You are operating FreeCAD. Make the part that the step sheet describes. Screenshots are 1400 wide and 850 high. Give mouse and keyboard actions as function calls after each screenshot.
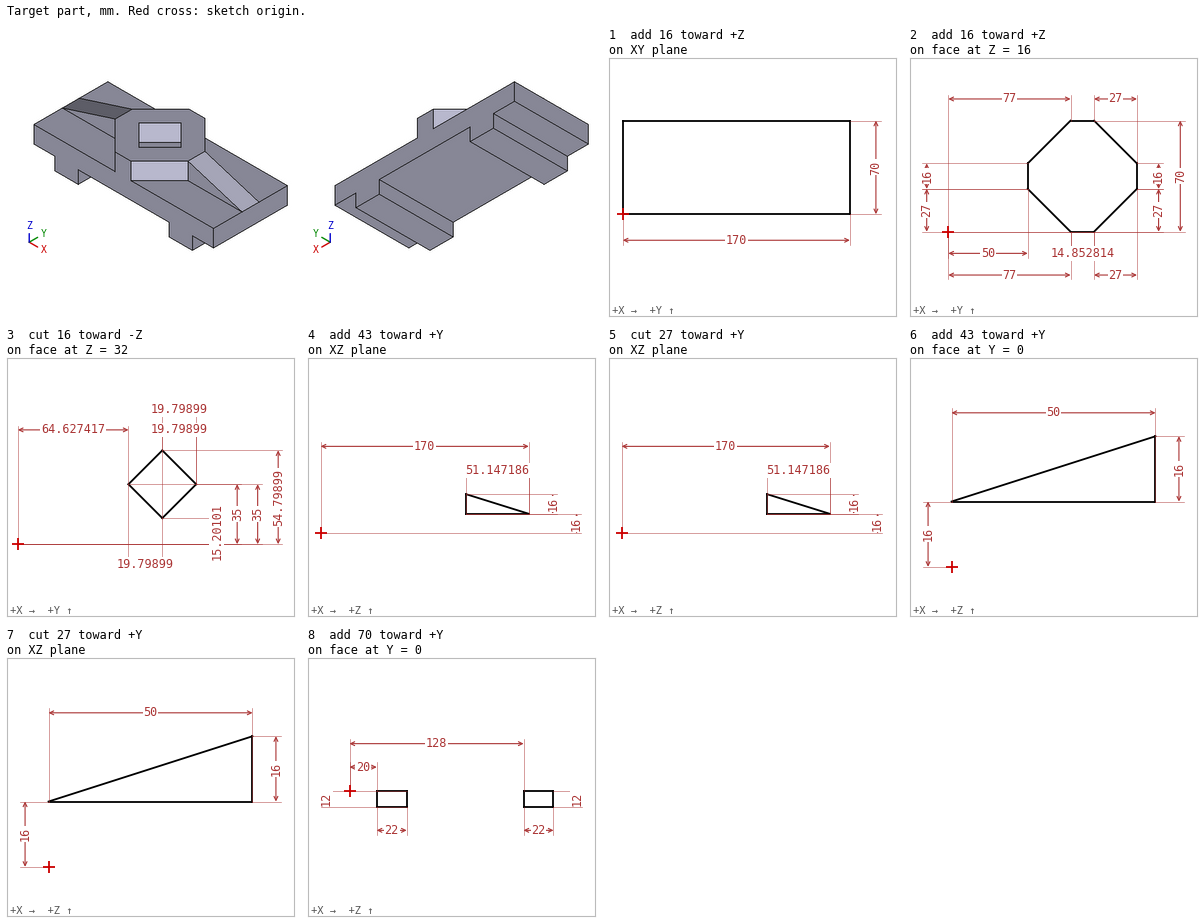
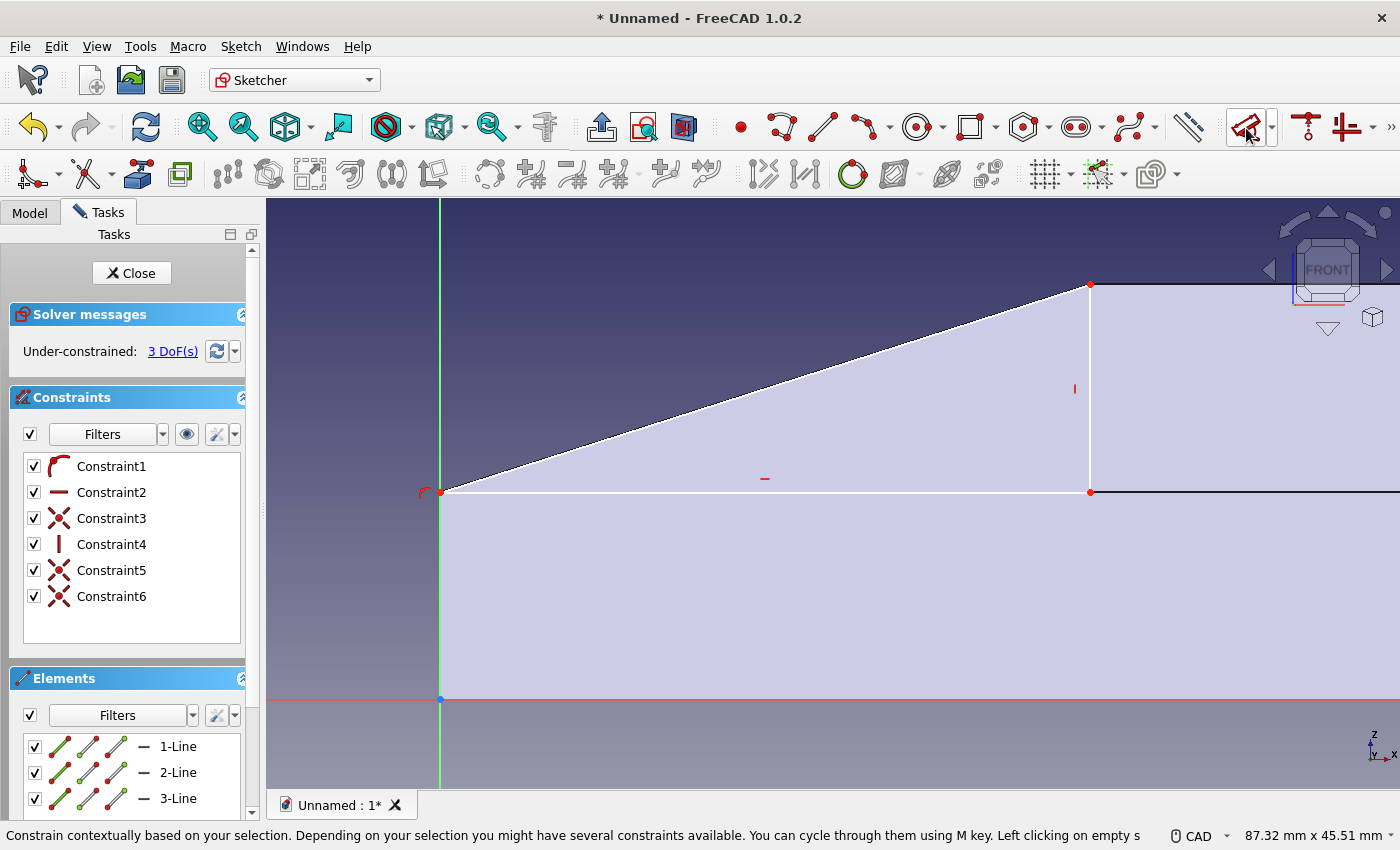
click(635, 493)
click(765, 527)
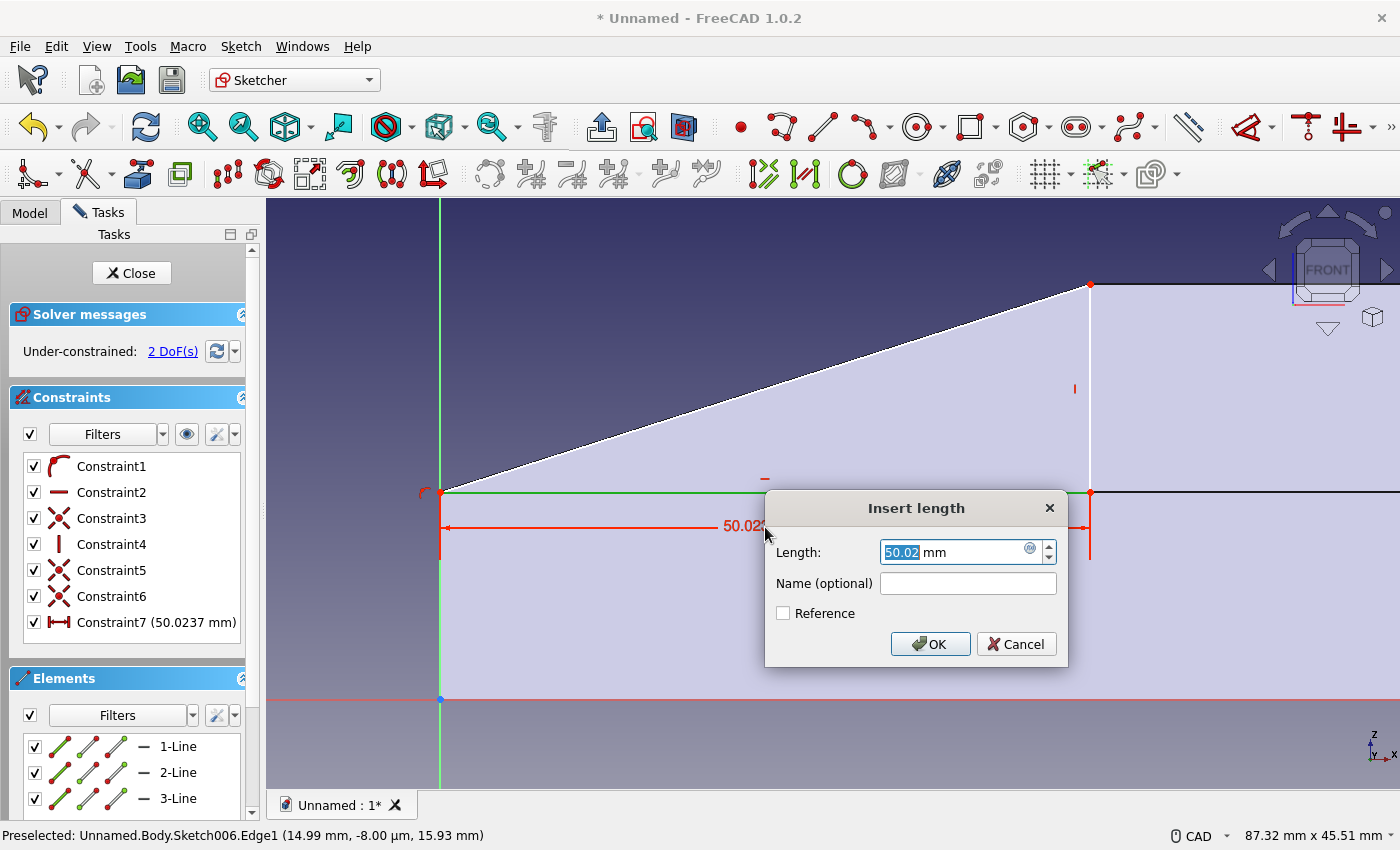
text(50)
key(Return)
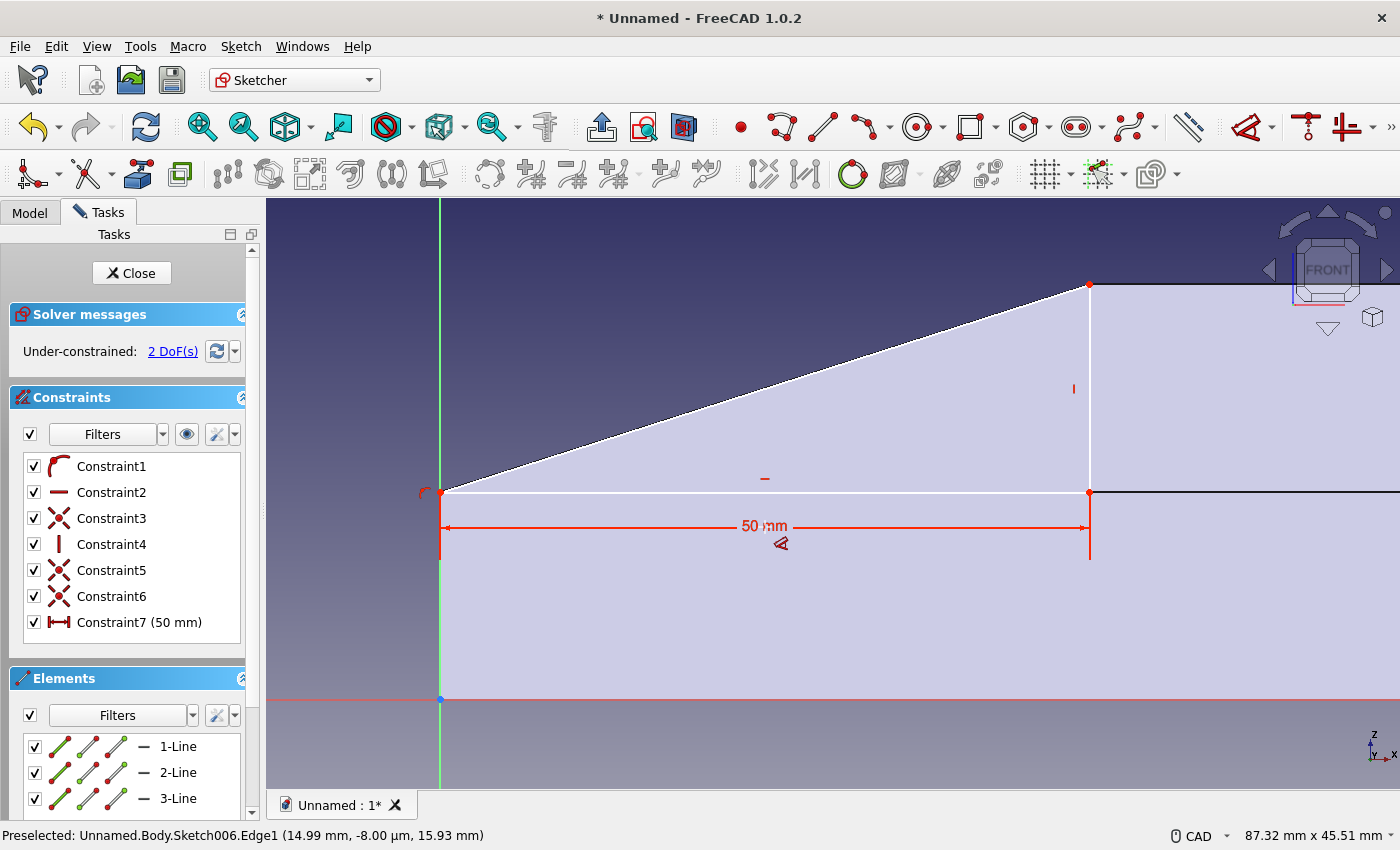
click(1090, 431)
click(1124, 389)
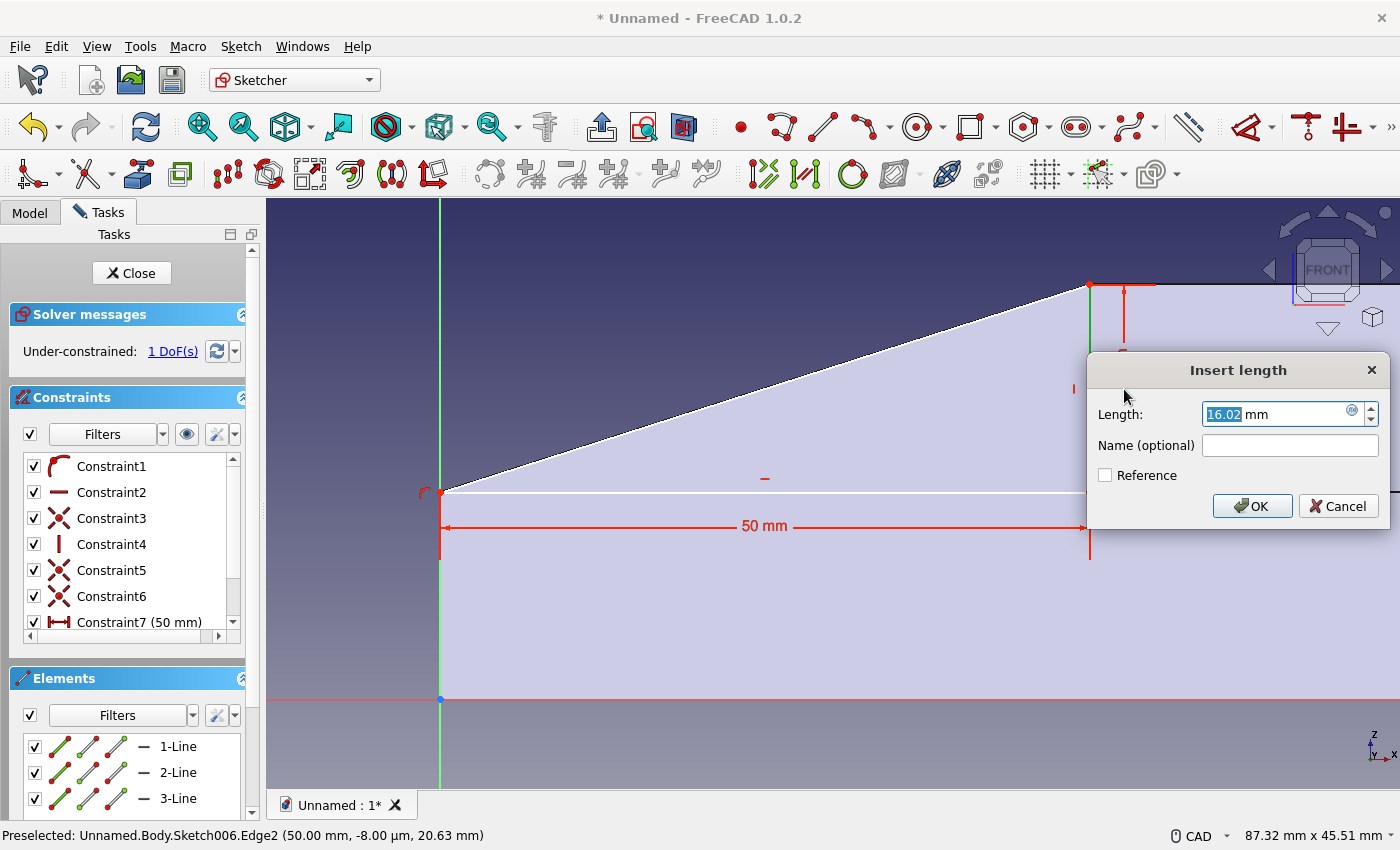
text(16)
key(Return)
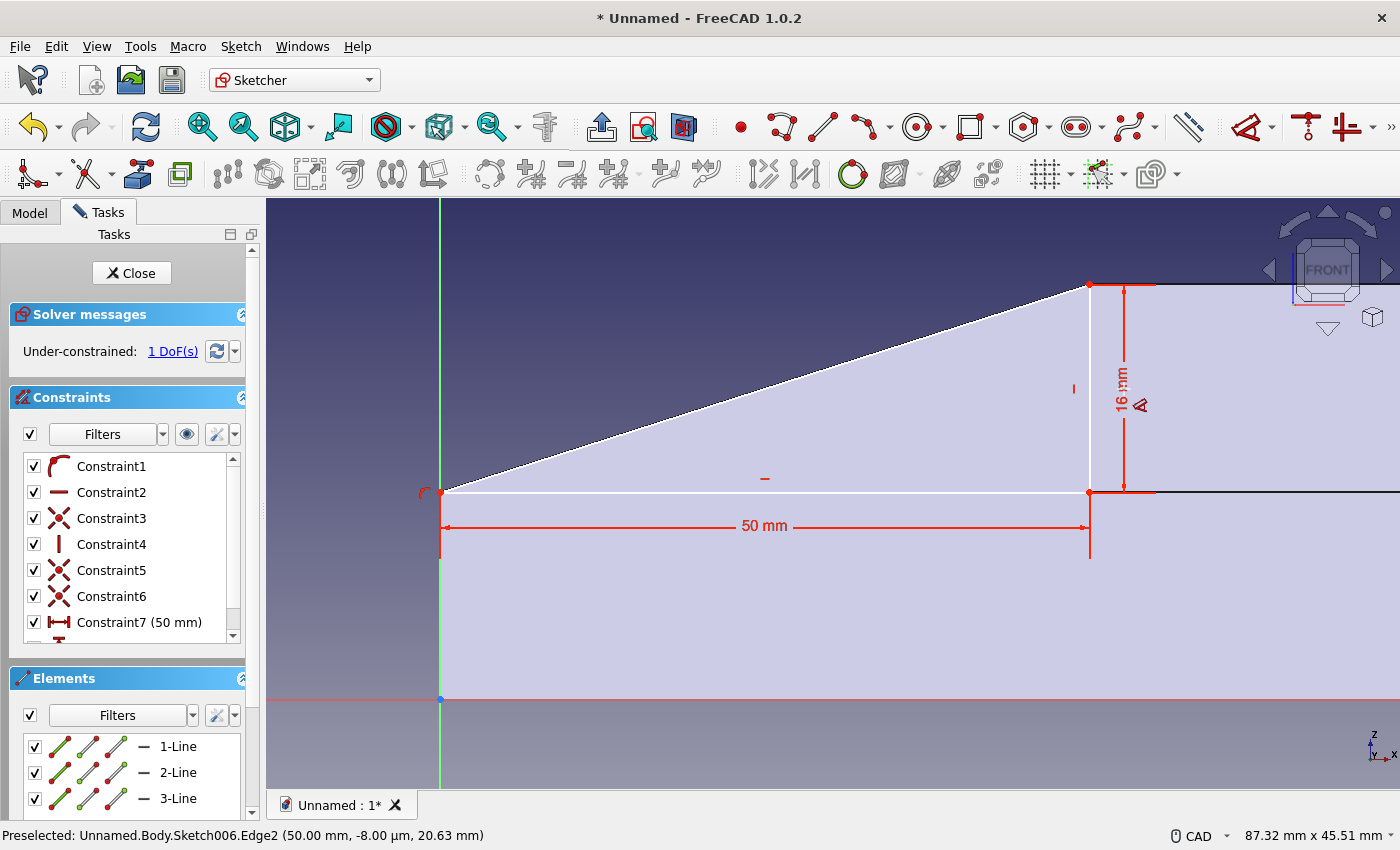
click(440, 493)
click(406, 596)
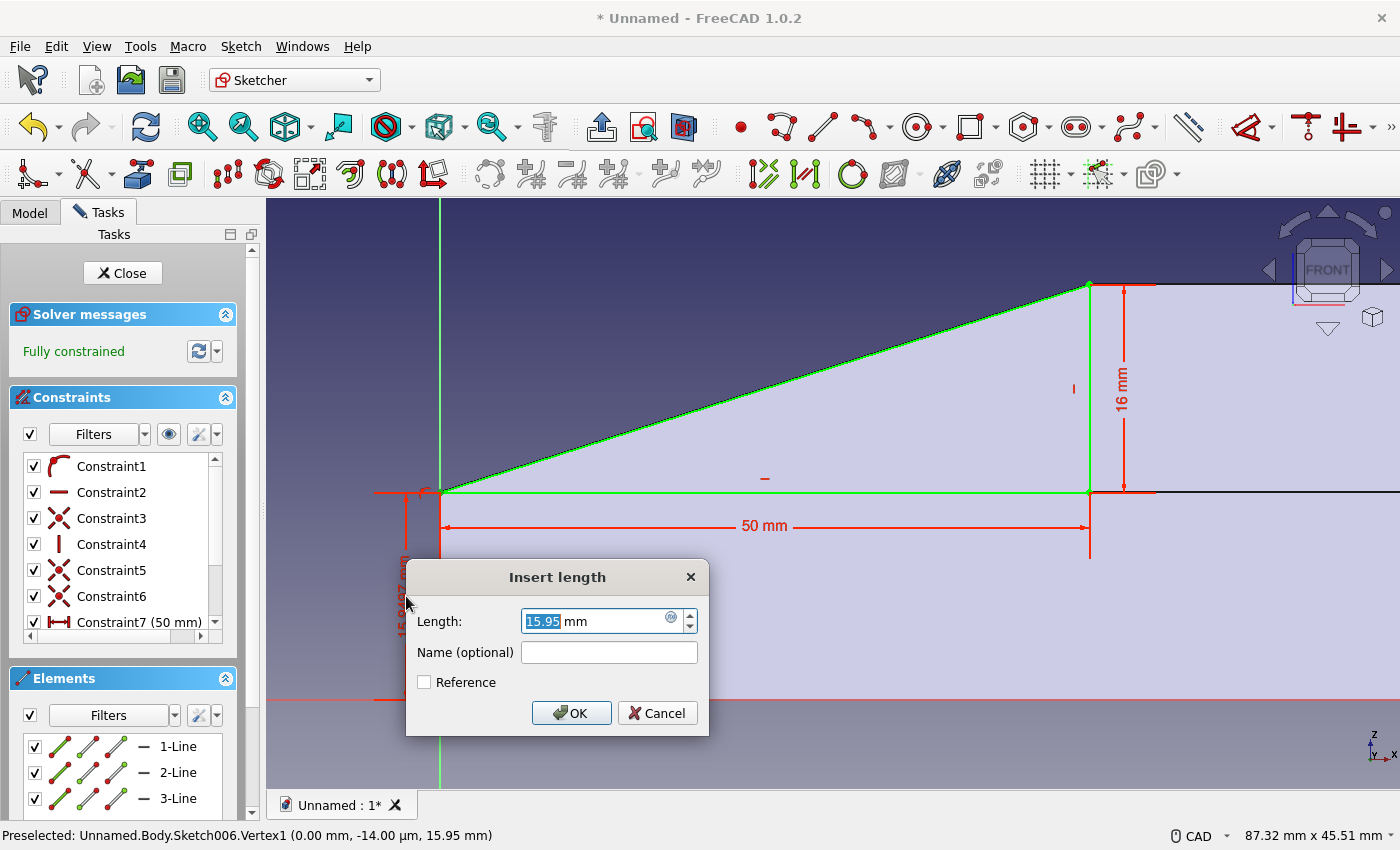
text(16)
key(Return)
key(Escape)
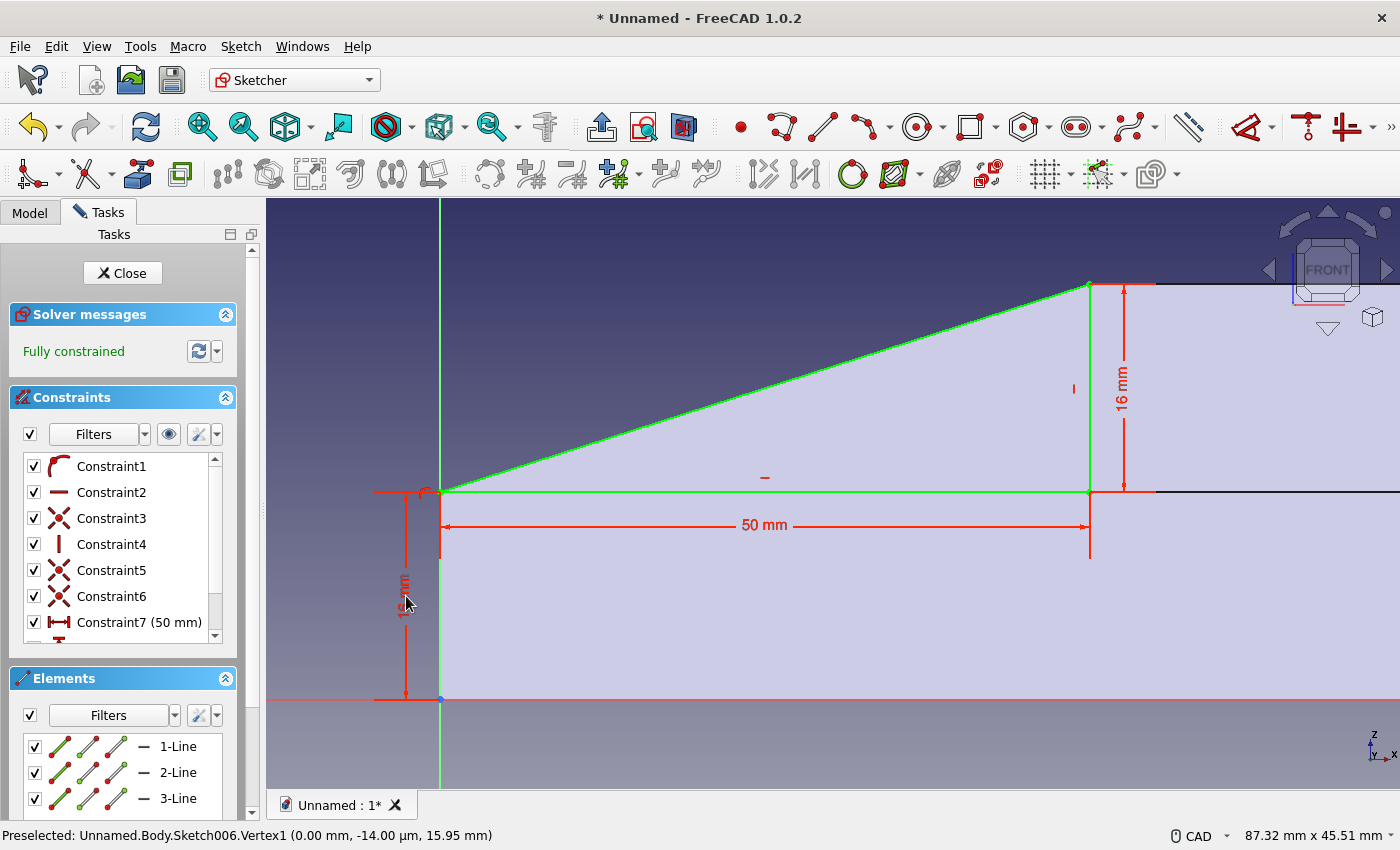
click(123, 273)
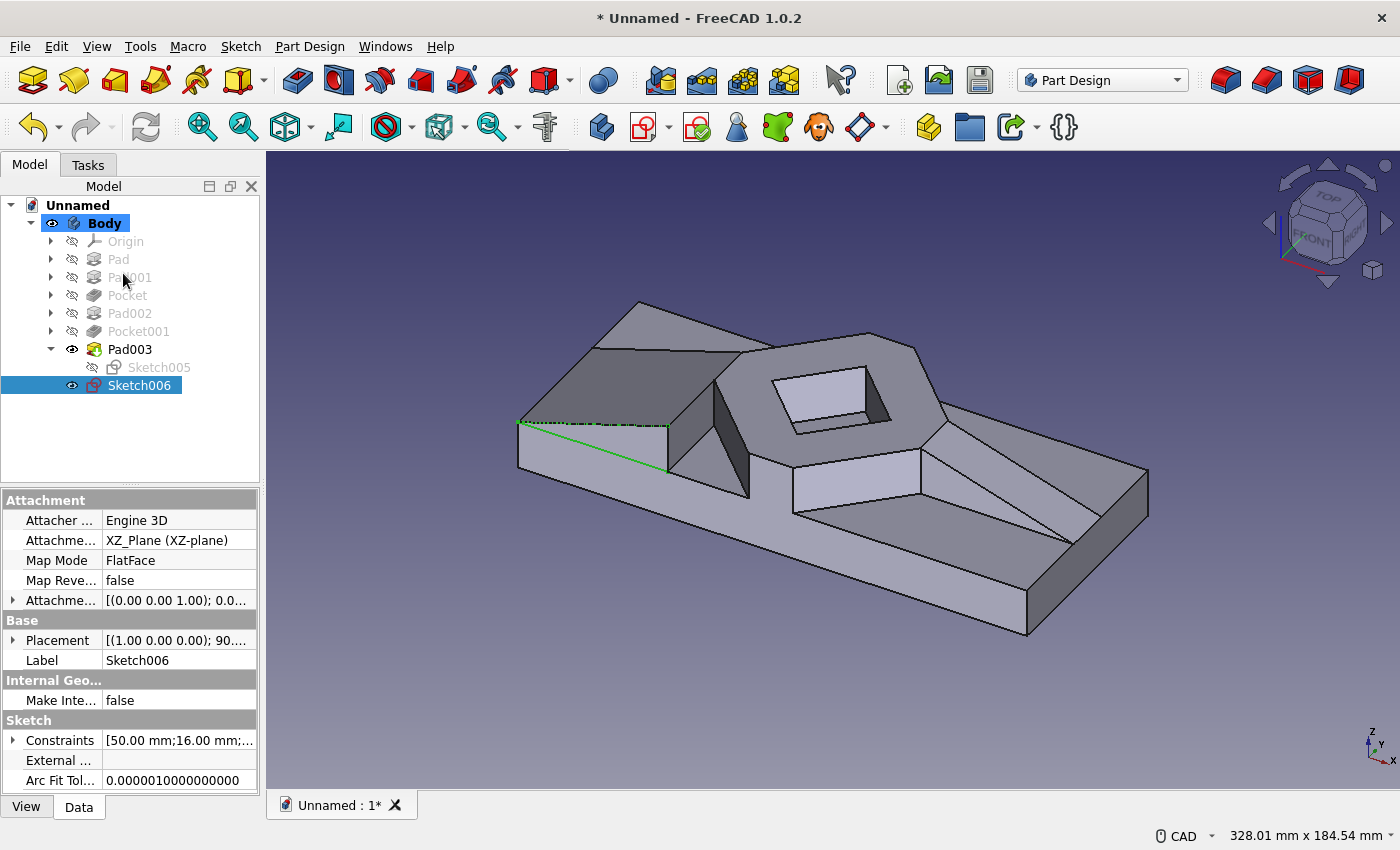
click(298, 80)